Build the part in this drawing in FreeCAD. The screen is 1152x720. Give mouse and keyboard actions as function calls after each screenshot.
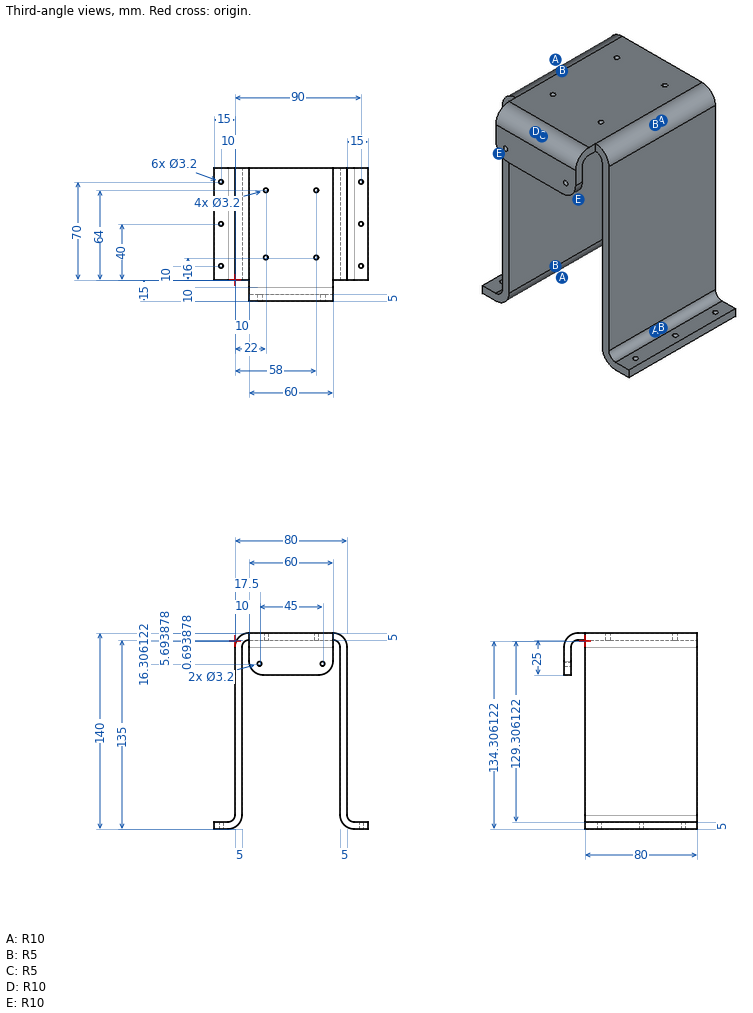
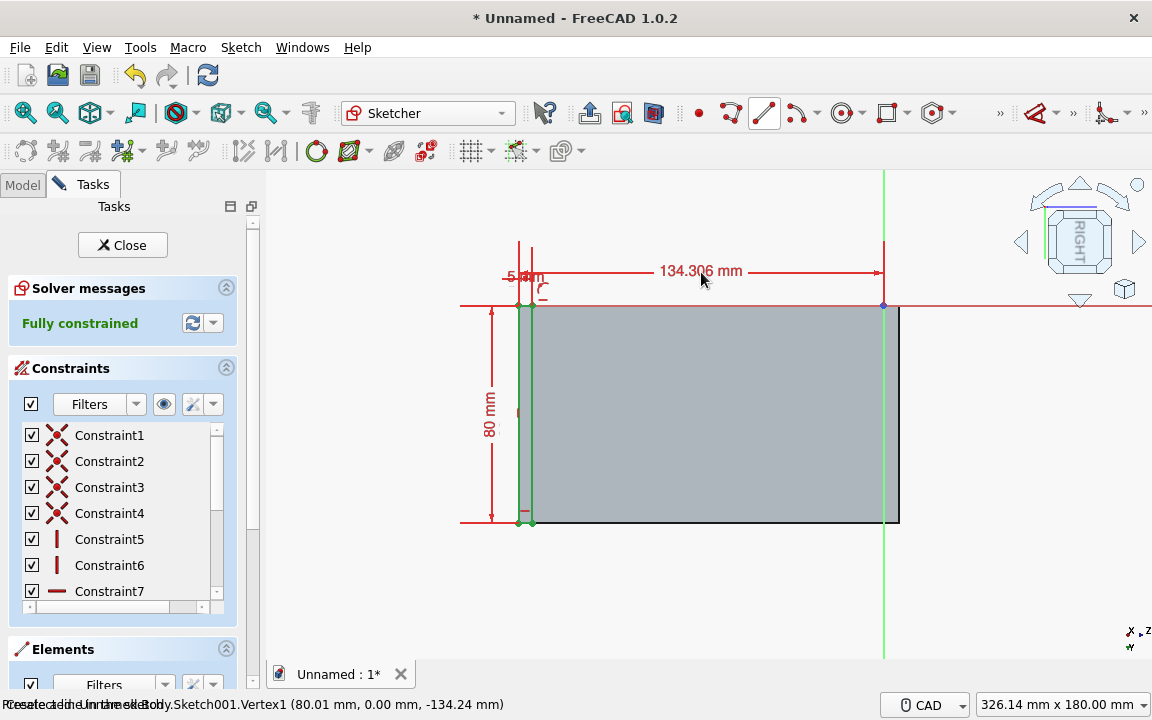
click(123, 245)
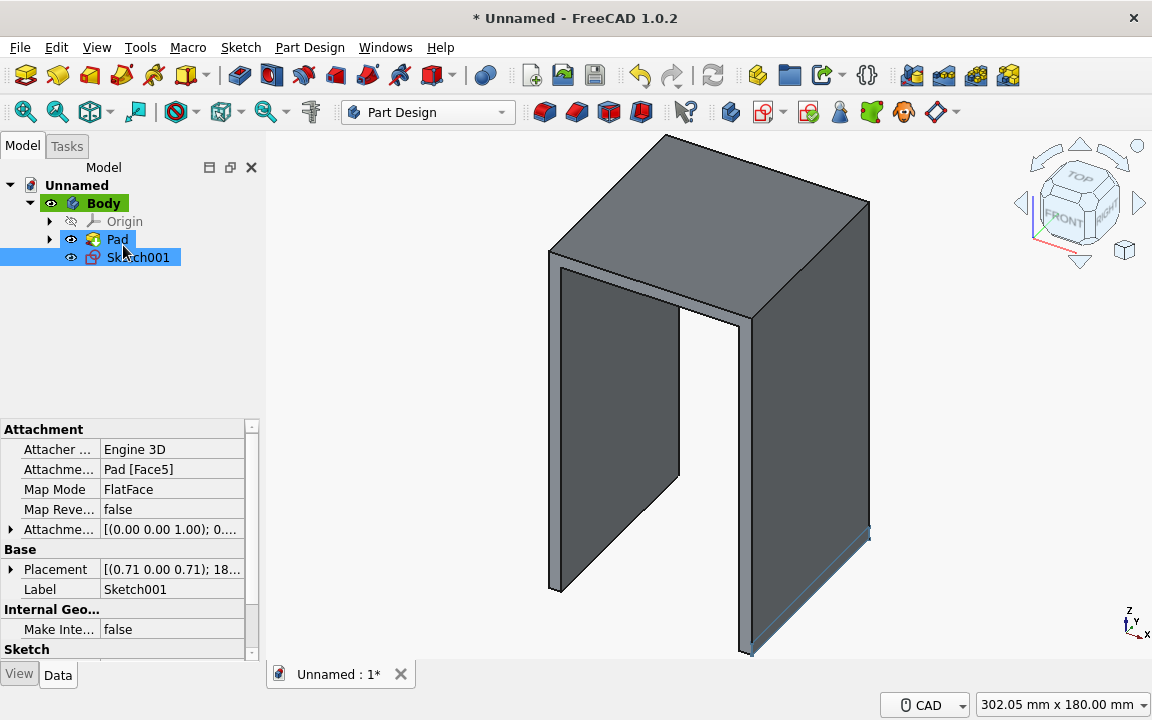
click(26, 76)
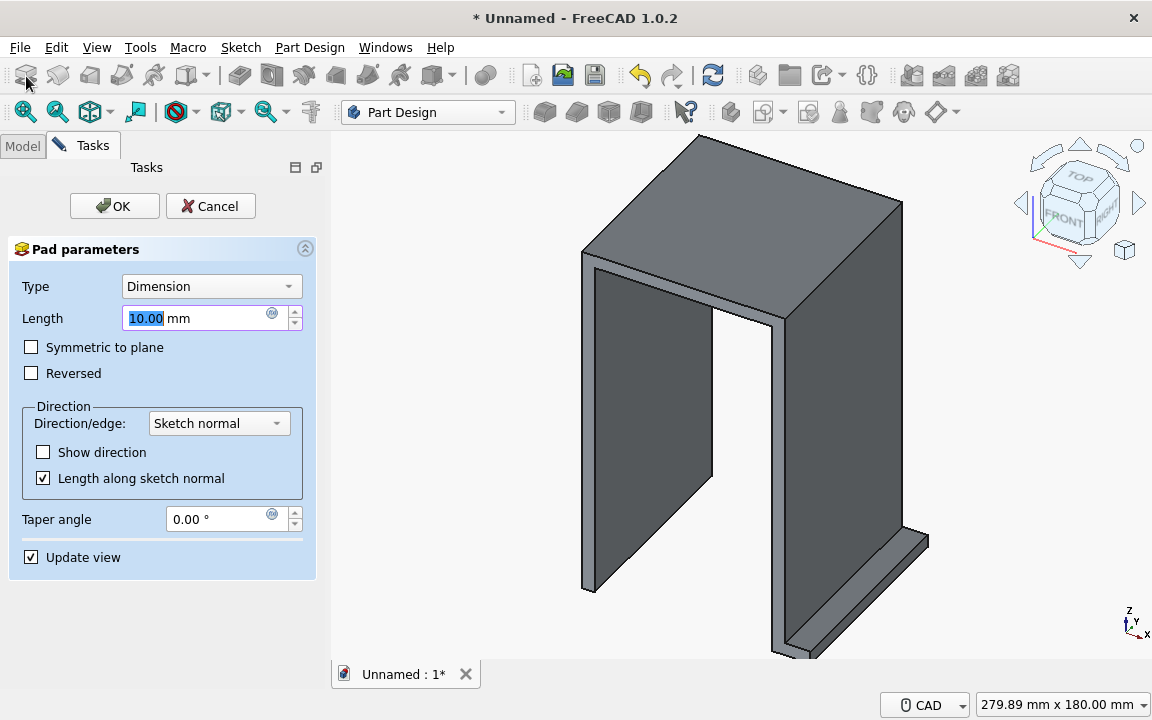
text(15)
key(Tab)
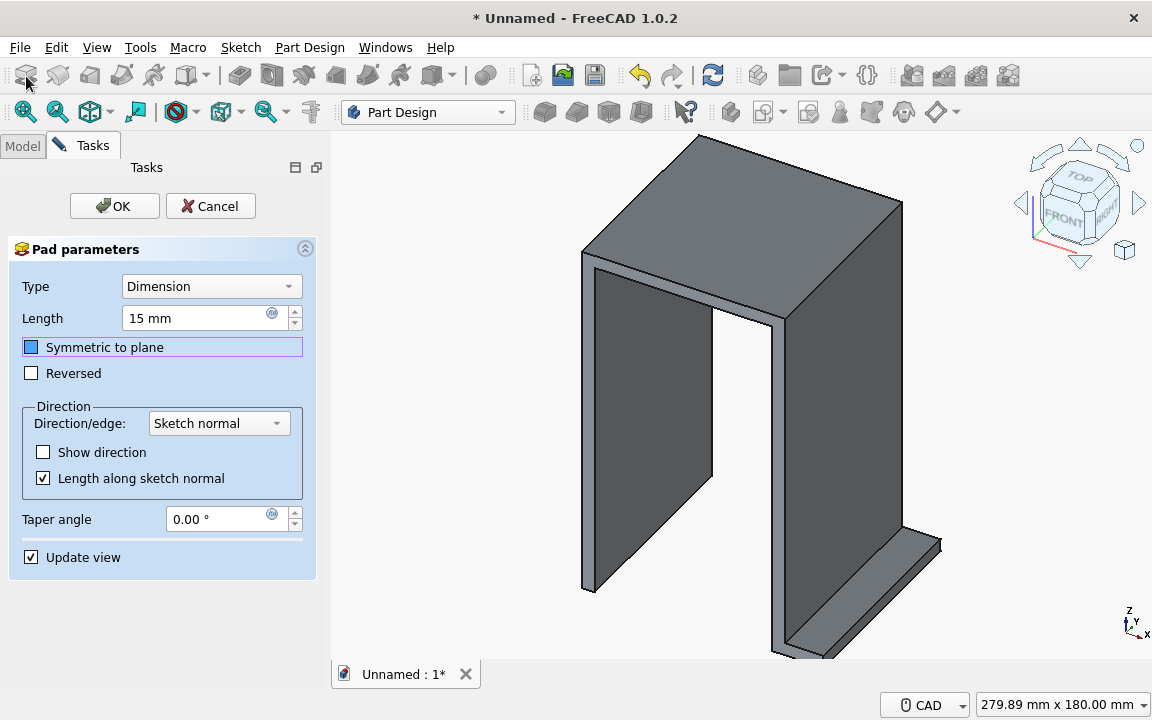
click(115, 206)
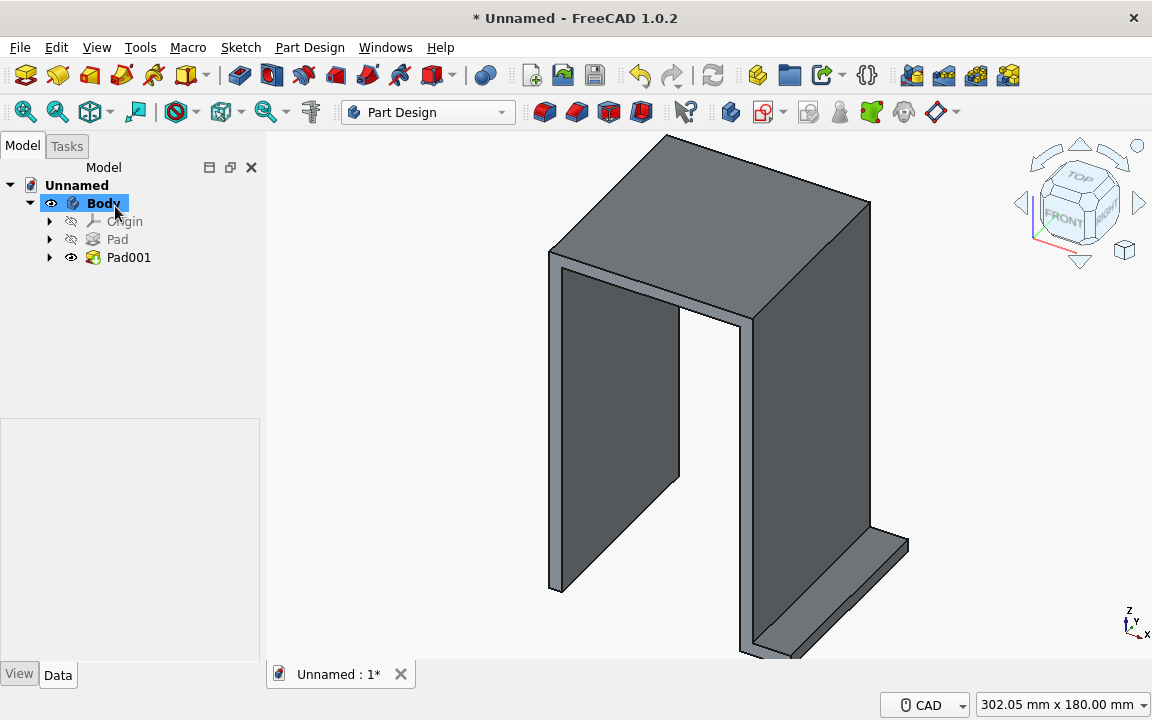
click(26, 112)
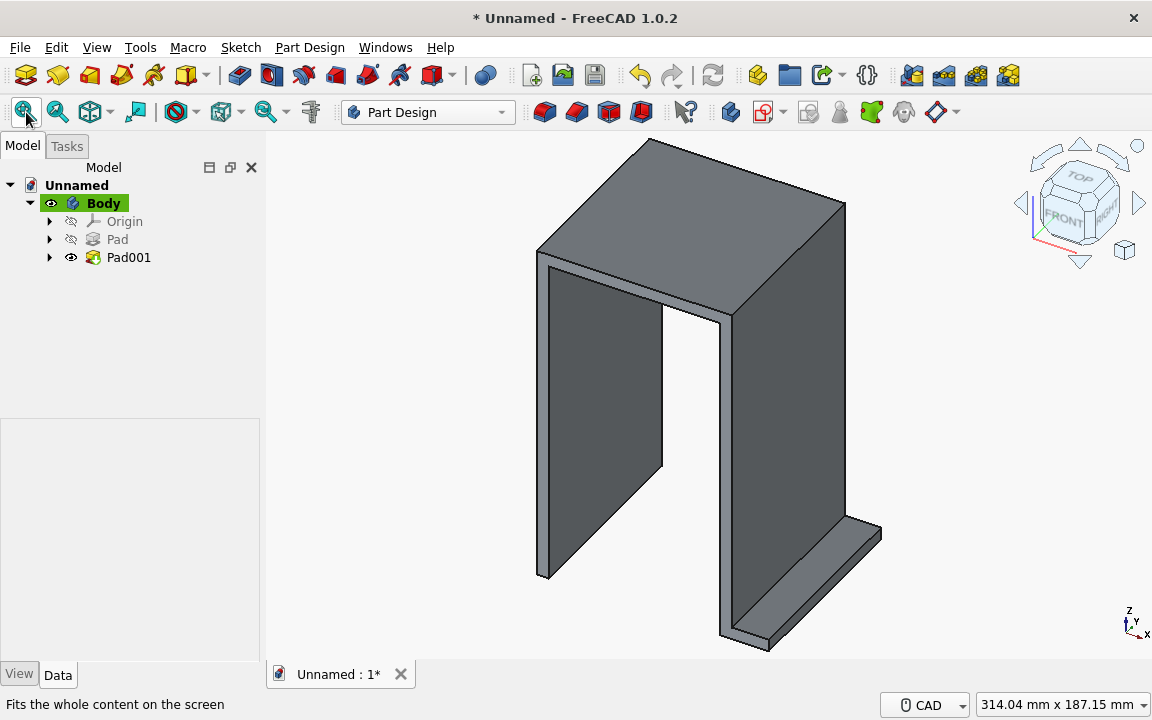
click(764, 112)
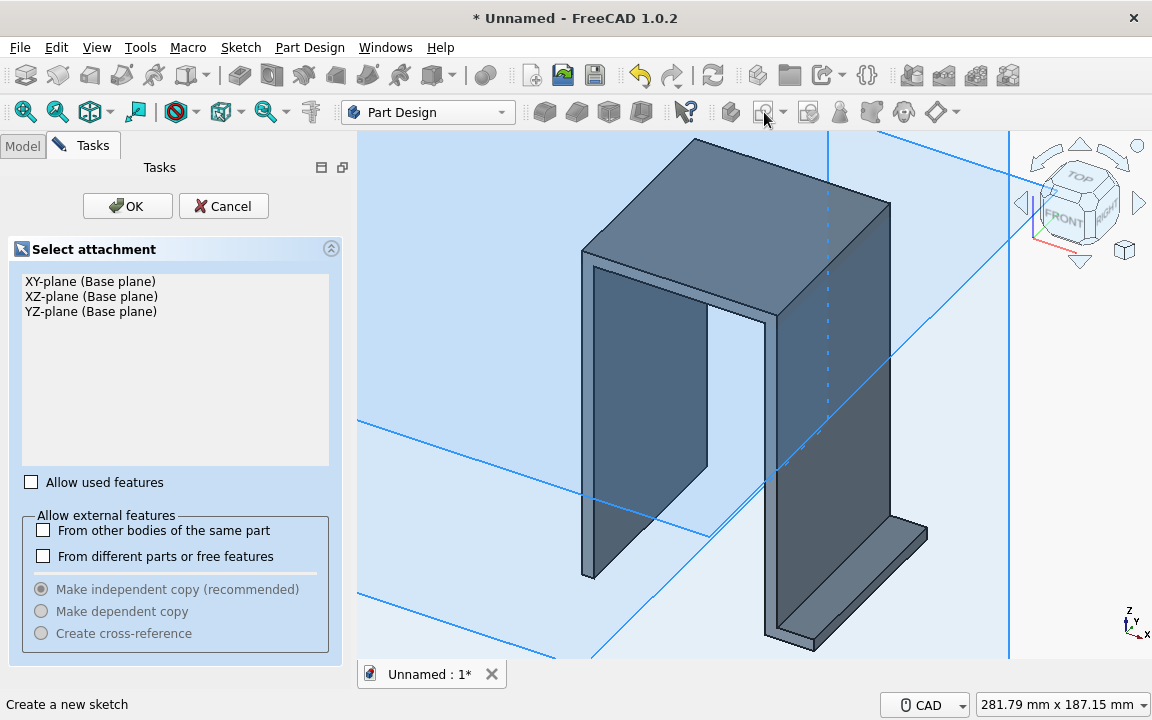
click(82, 312)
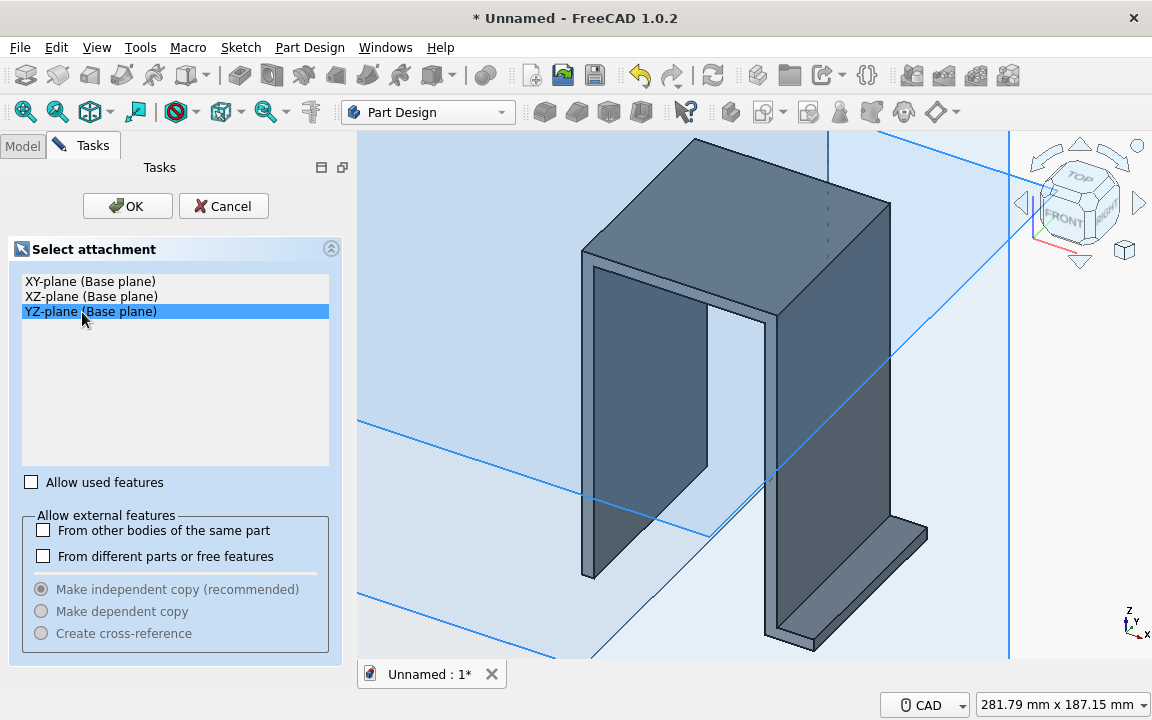
click(128, 206)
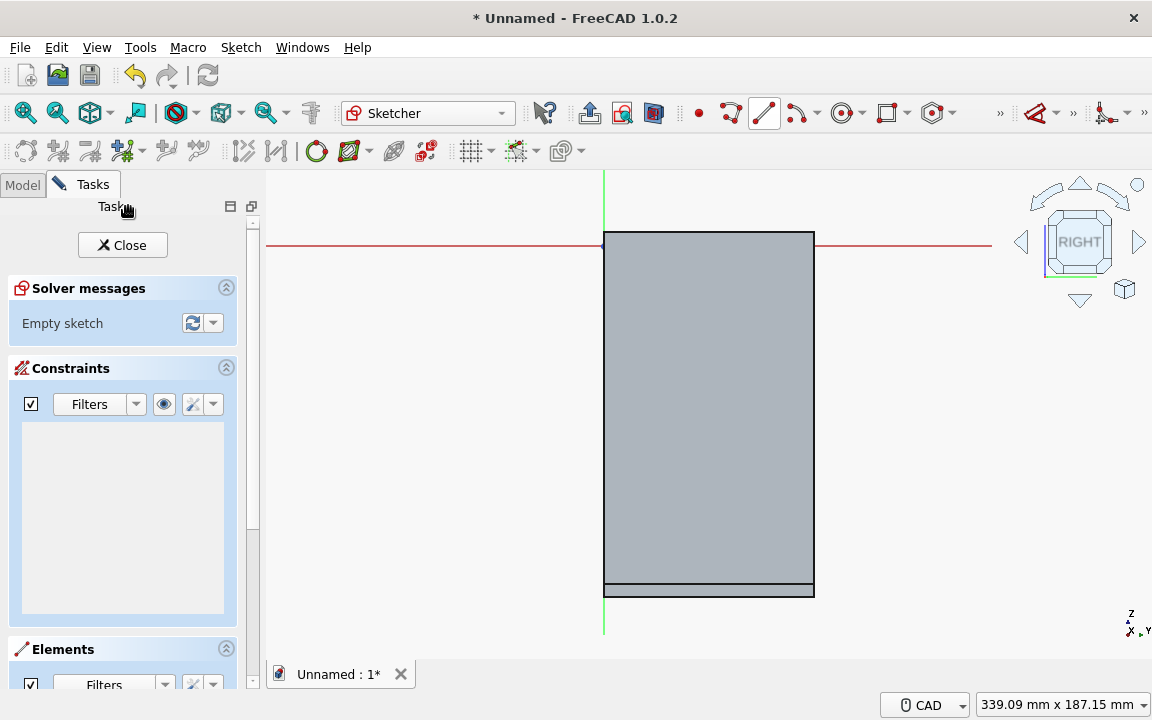
key(q)
key(s)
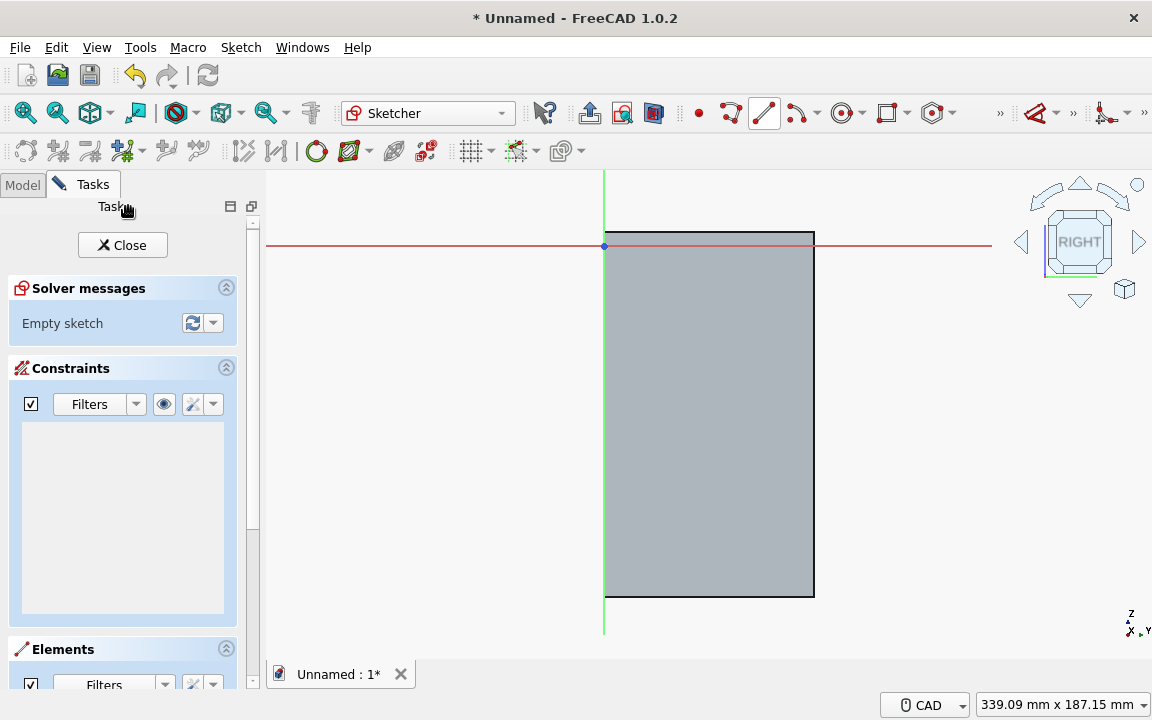
click(888, 114)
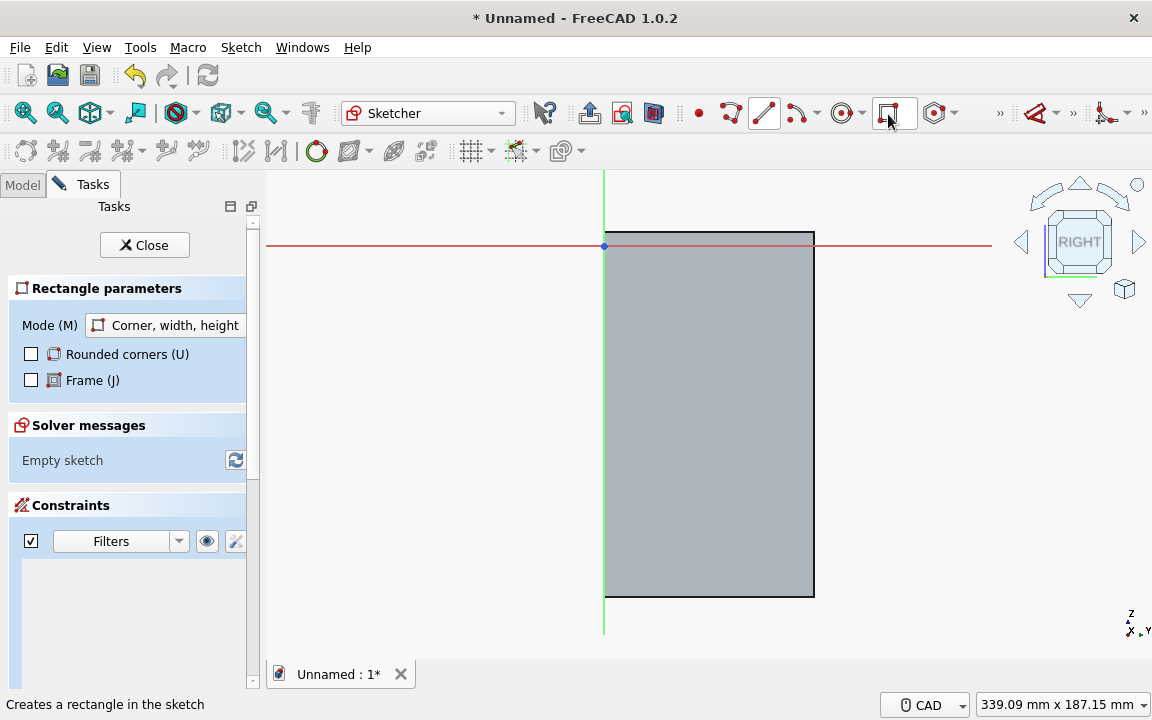
click(604, 584)
move(814, 597)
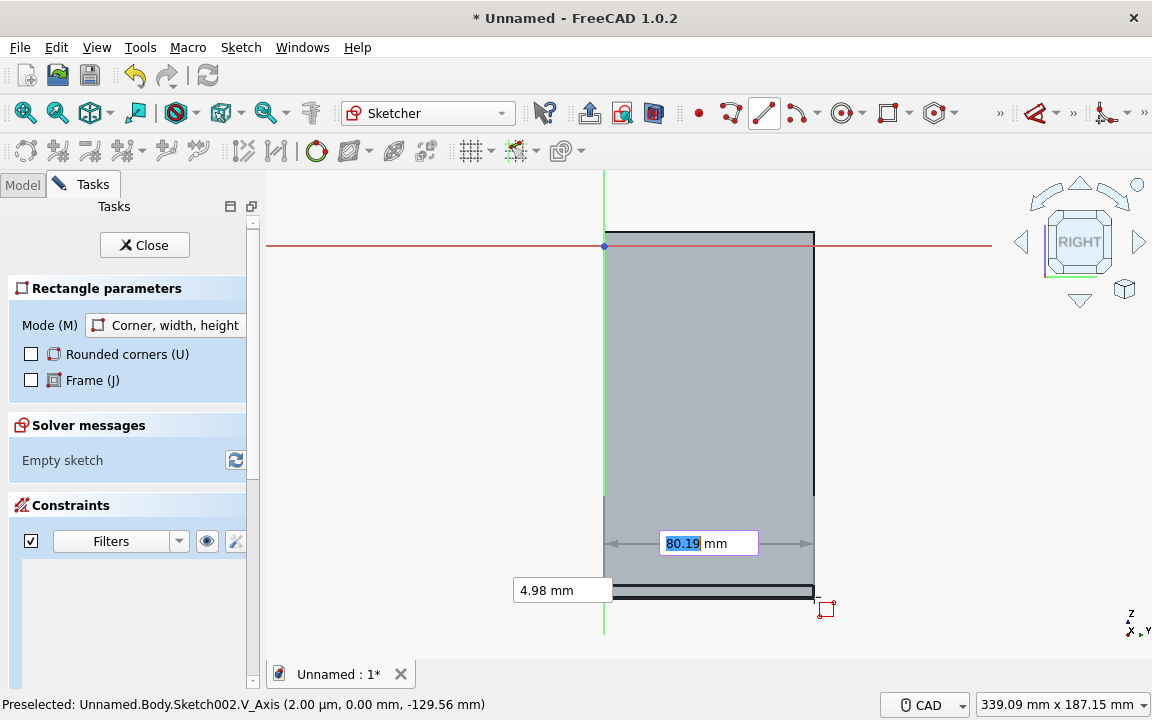
text(80)
key(Tab)
text(5)
key(Return)
key(Escape)